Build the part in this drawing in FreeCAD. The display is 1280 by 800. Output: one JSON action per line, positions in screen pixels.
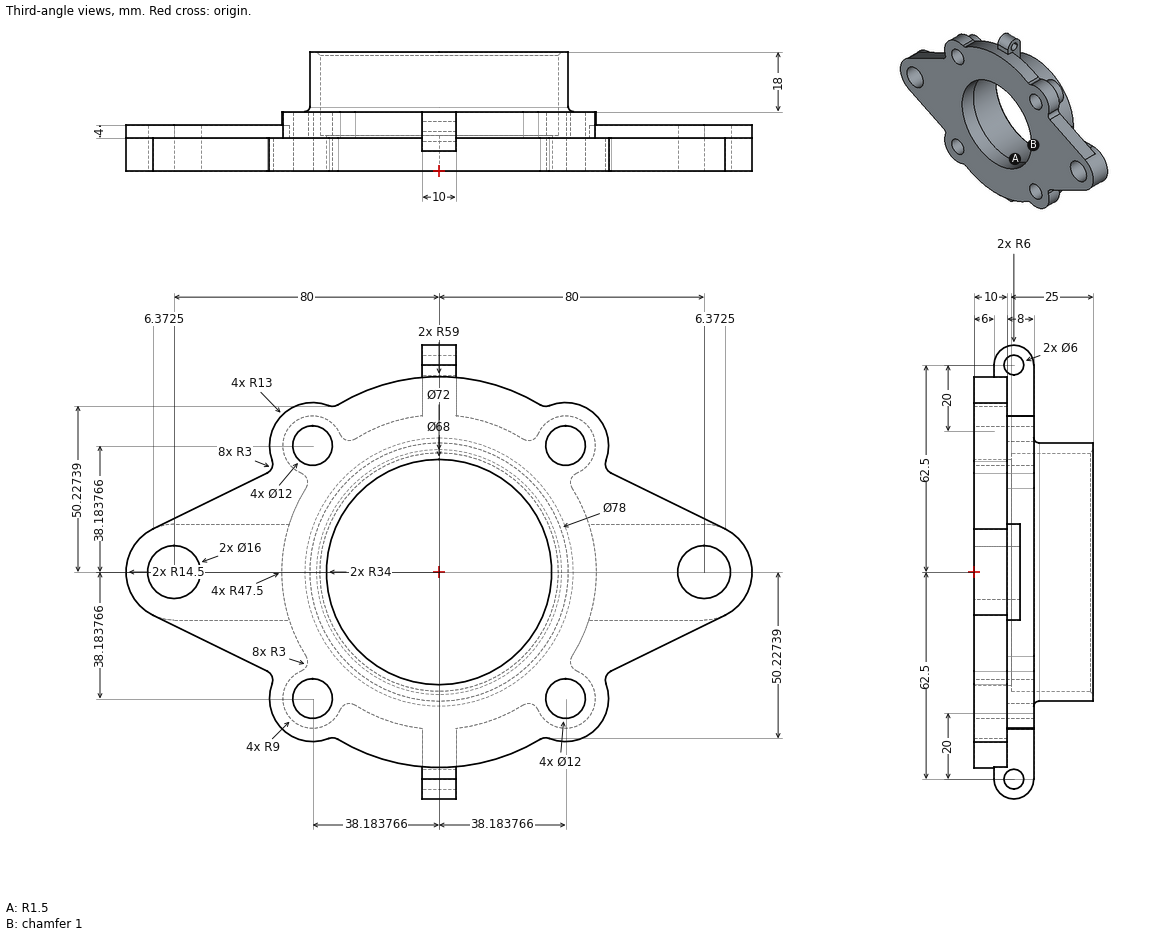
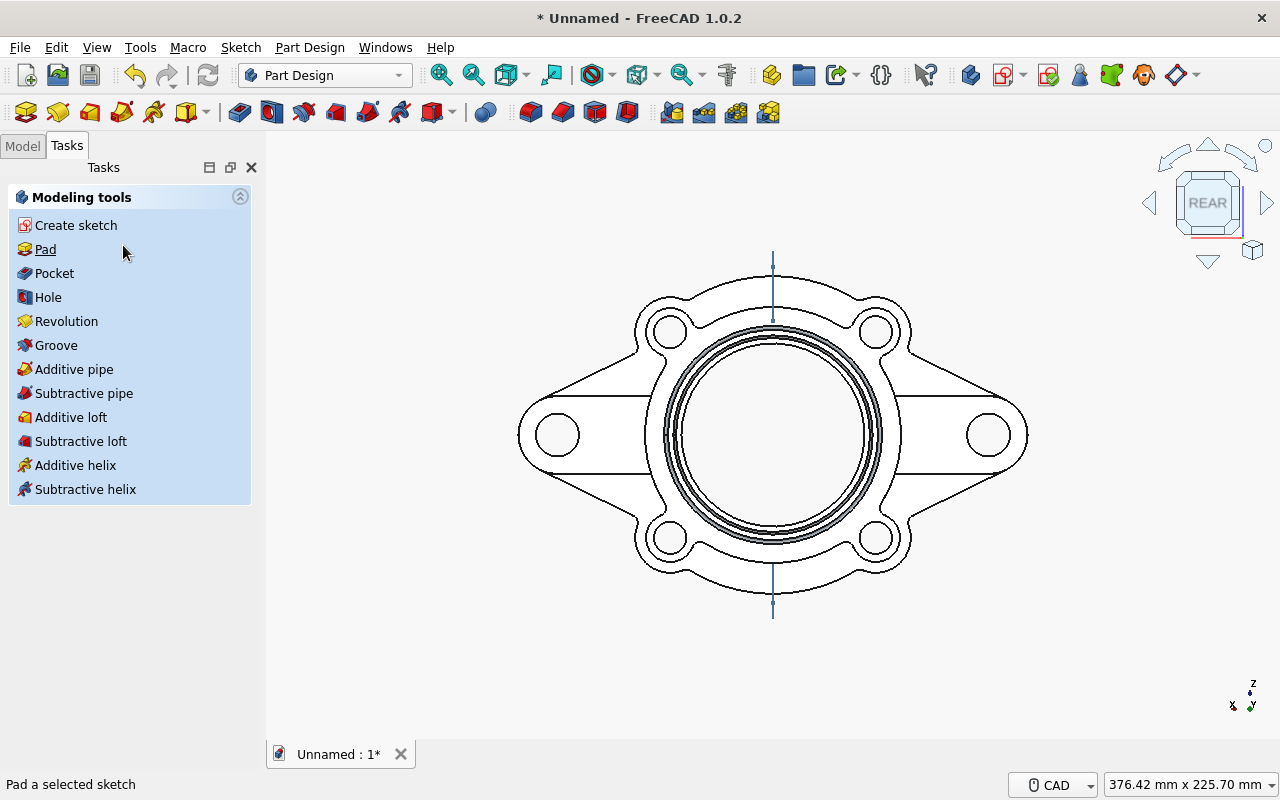
{"action": "left_click", "coordinate": [26, 112]}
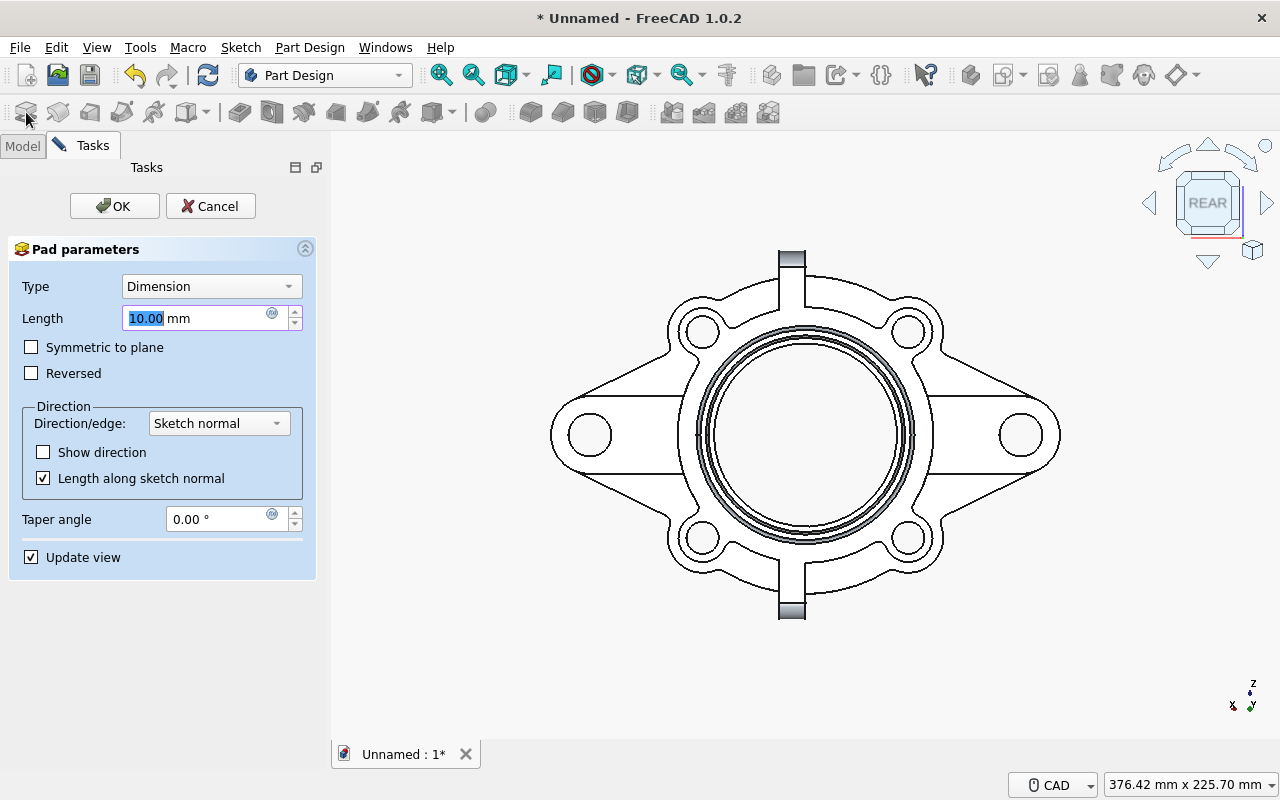
{"action": "type", "text": "10"}
{"action": "key", "text": "Tab"}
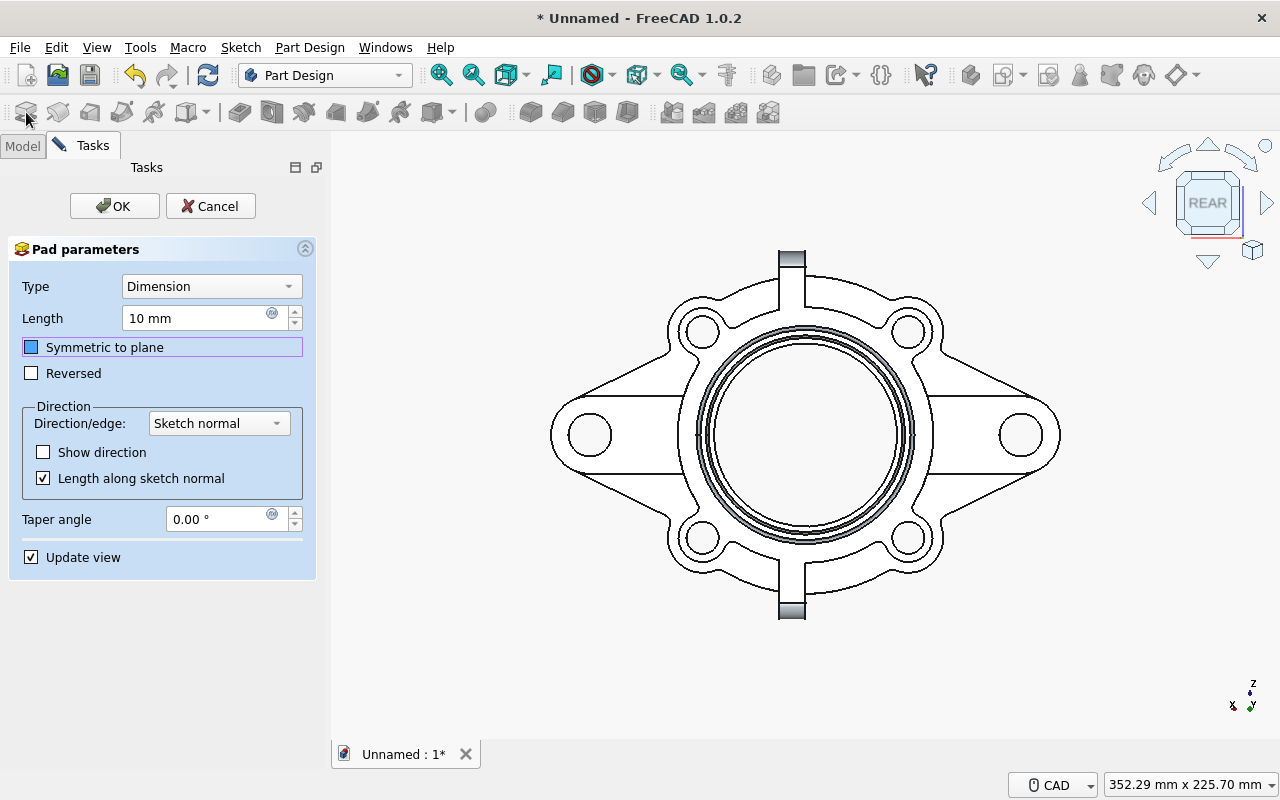
{"action": "left_click", "coordinate": [30, 347]}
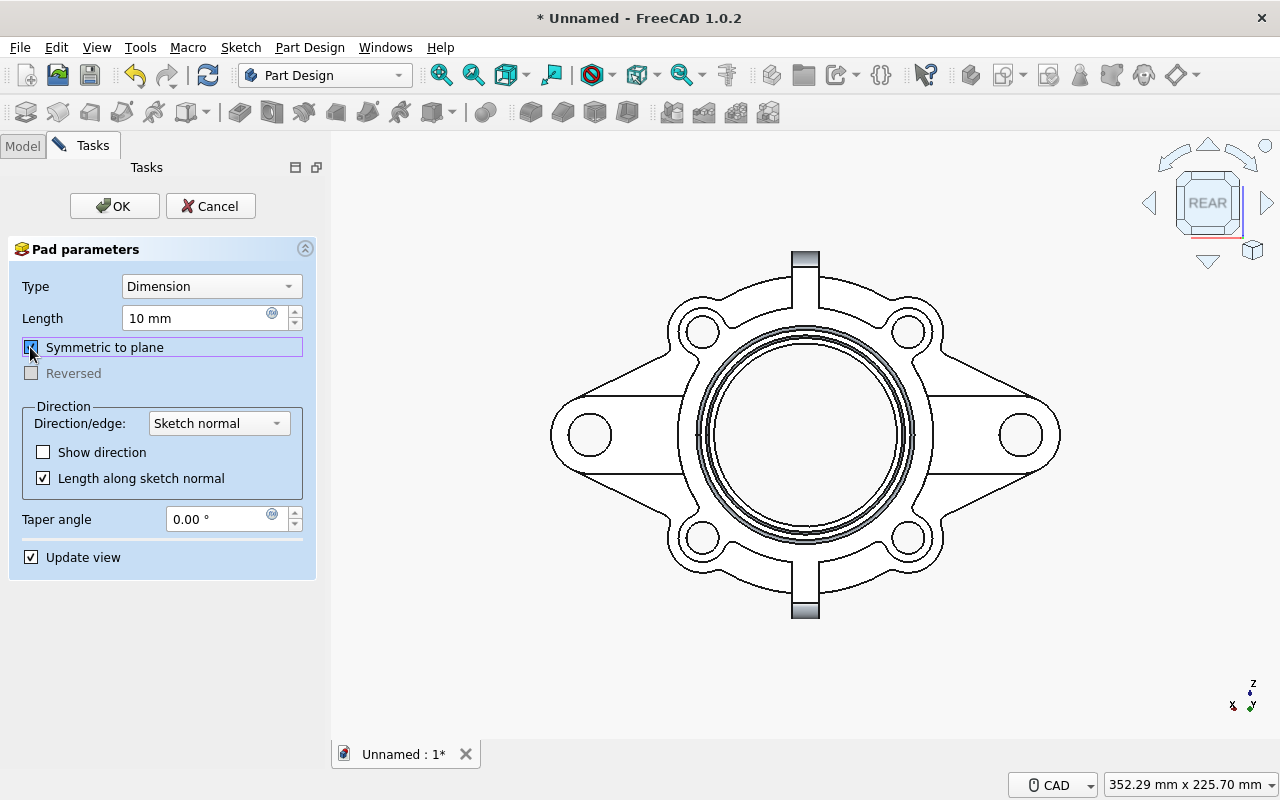
{"action": "left_click", "coordinate": [115, 206]}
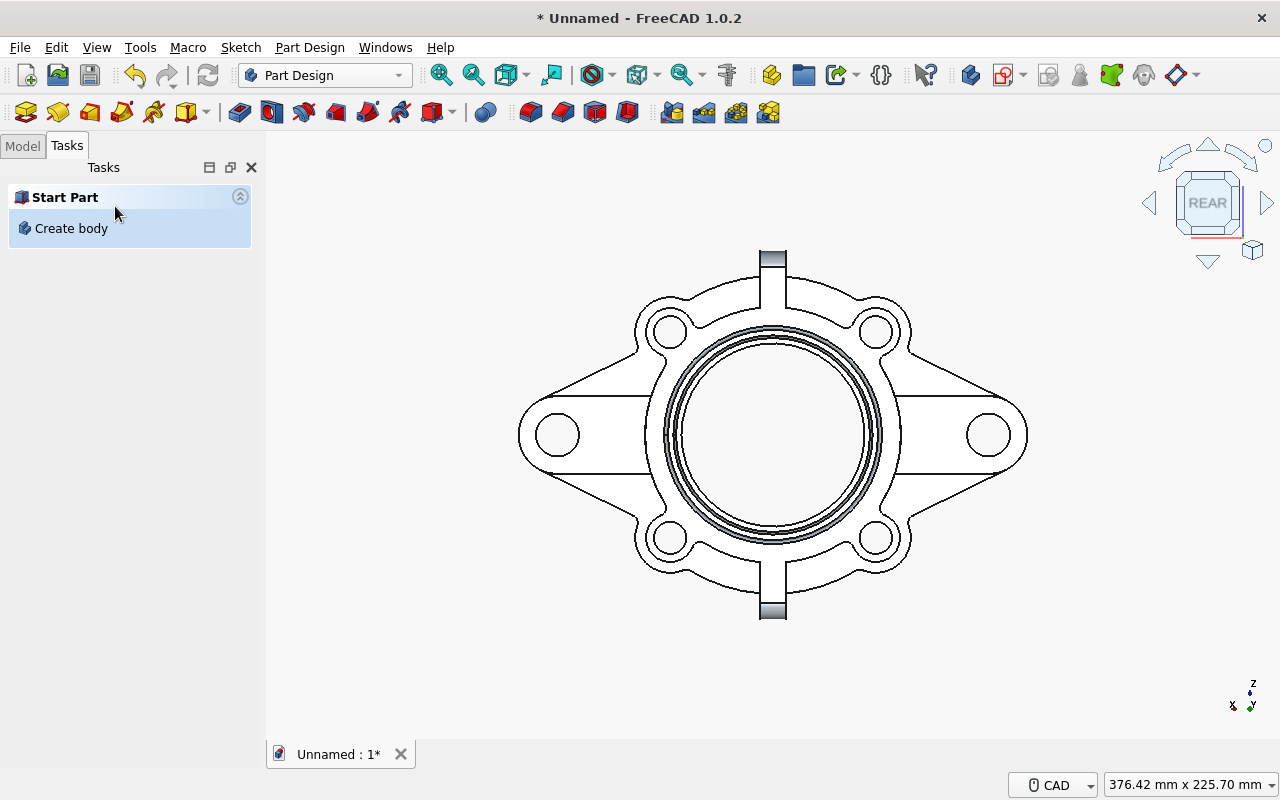
{"action": "key", "text": "0"}